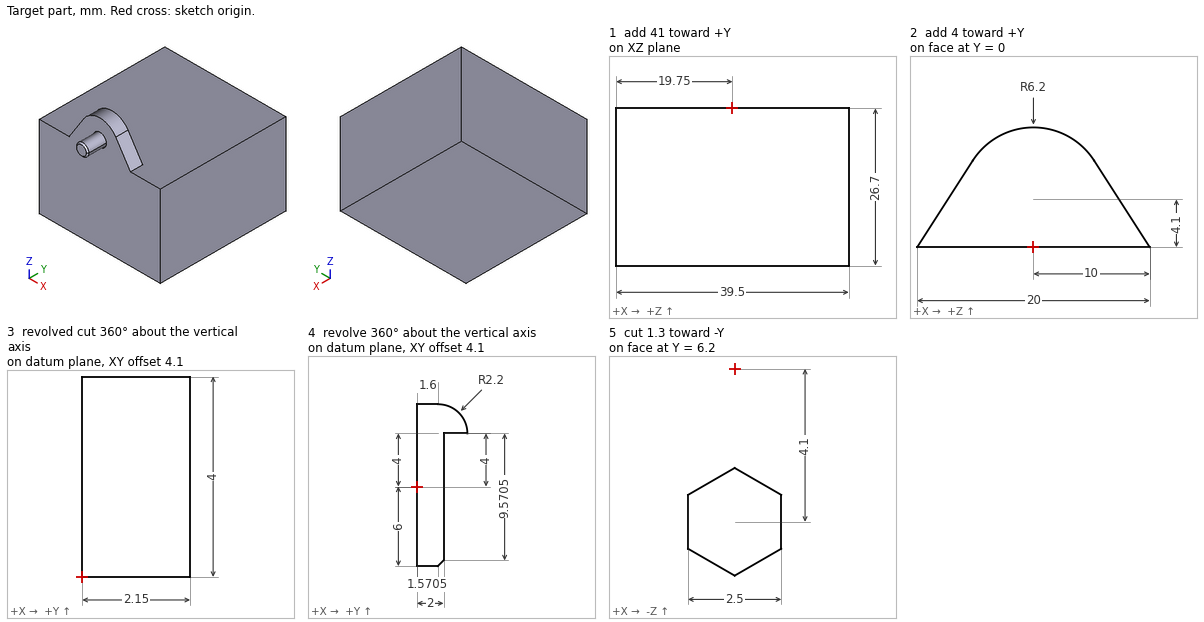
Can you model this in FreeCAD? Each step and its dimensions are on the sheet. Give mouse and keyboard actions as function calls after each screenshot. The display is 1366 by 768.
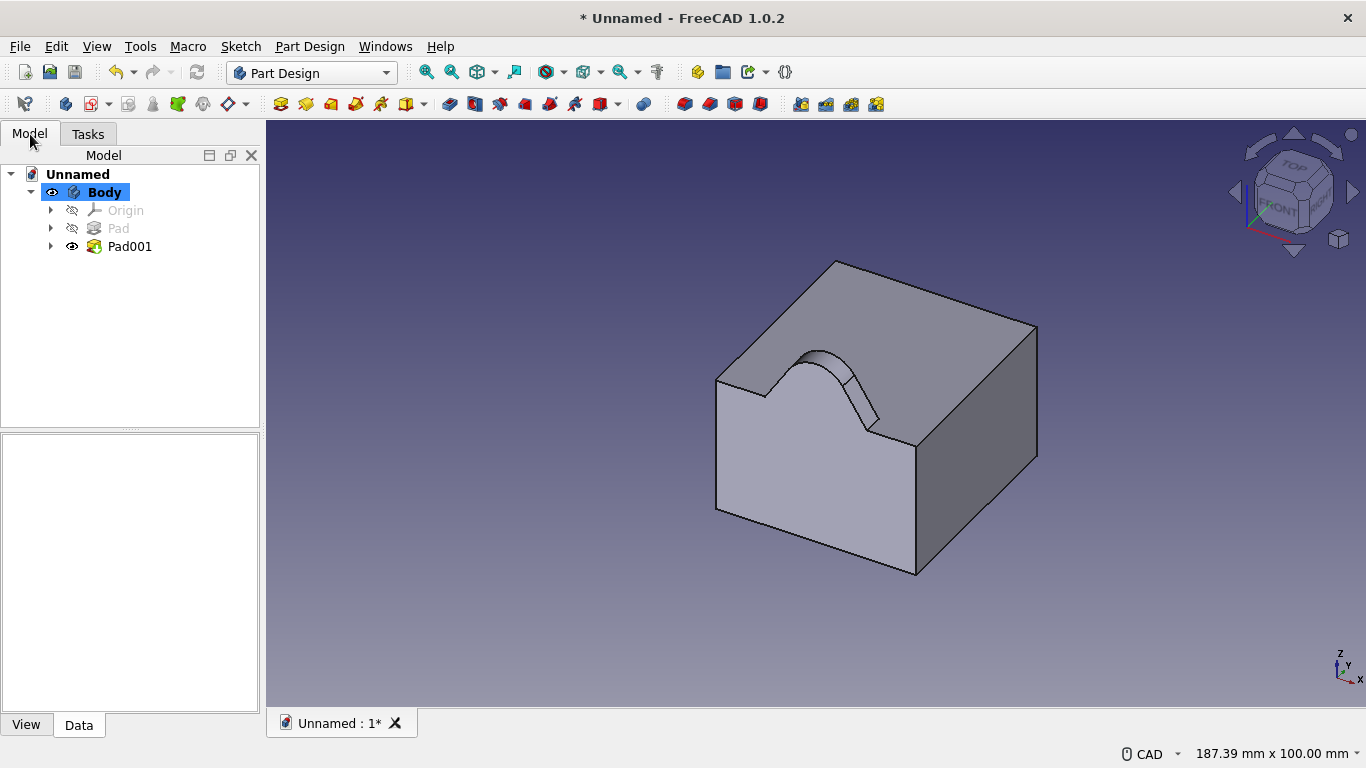
click(51, 210)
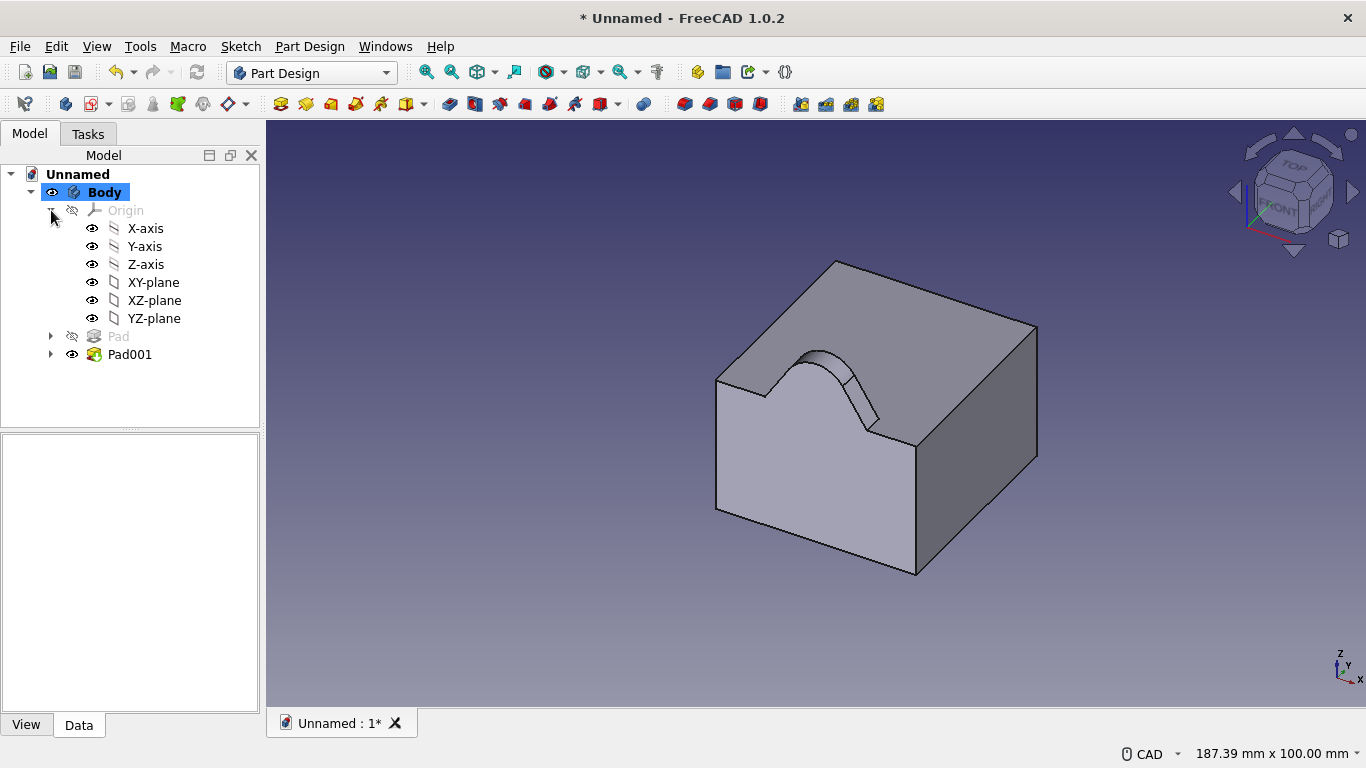
click(137, 282)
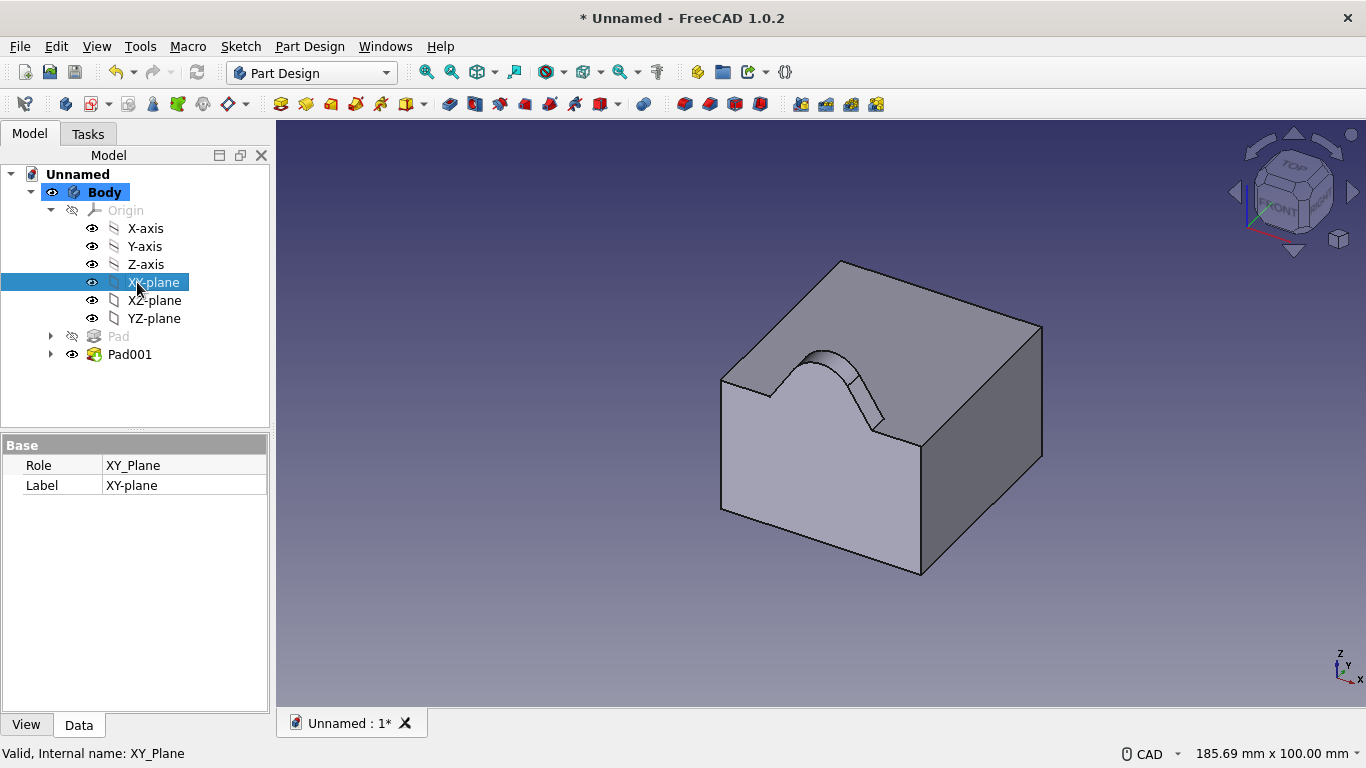
click(228, 104)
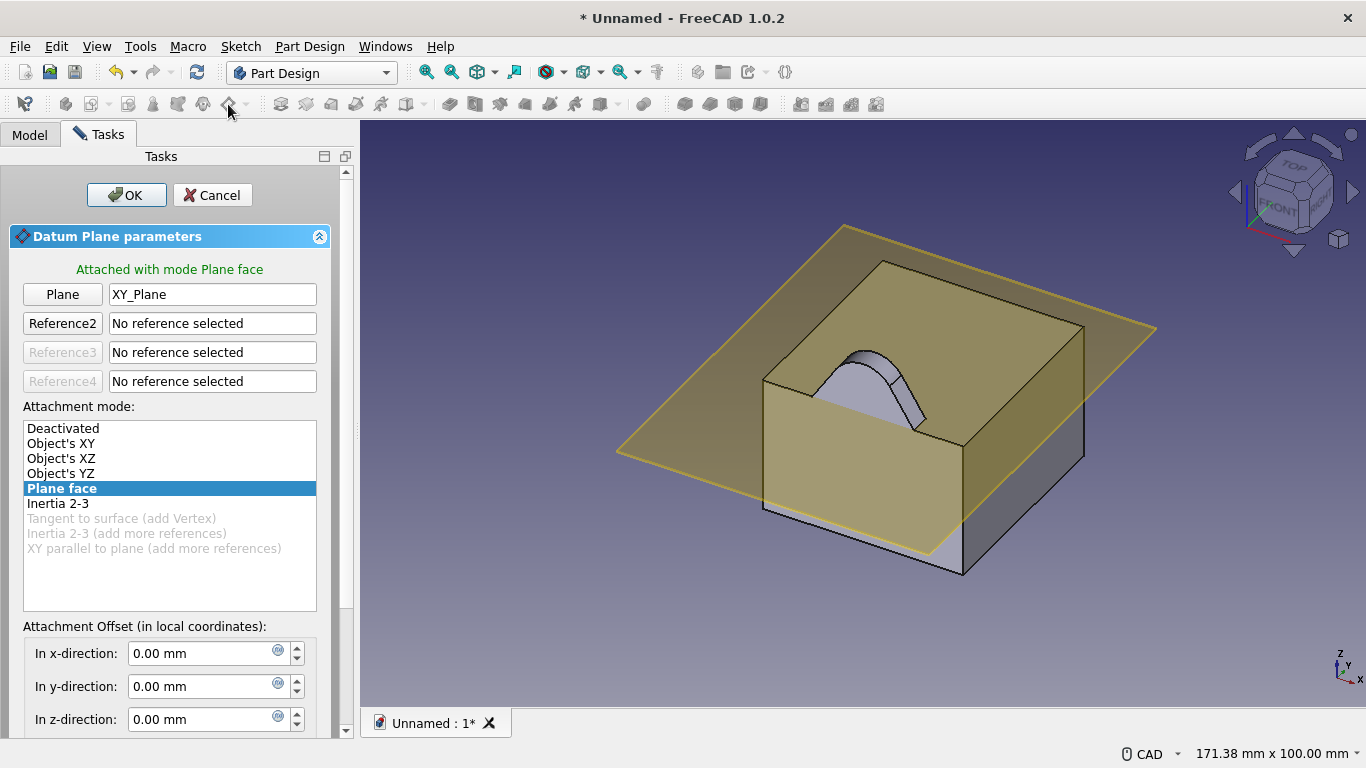
triple_click(210, 720)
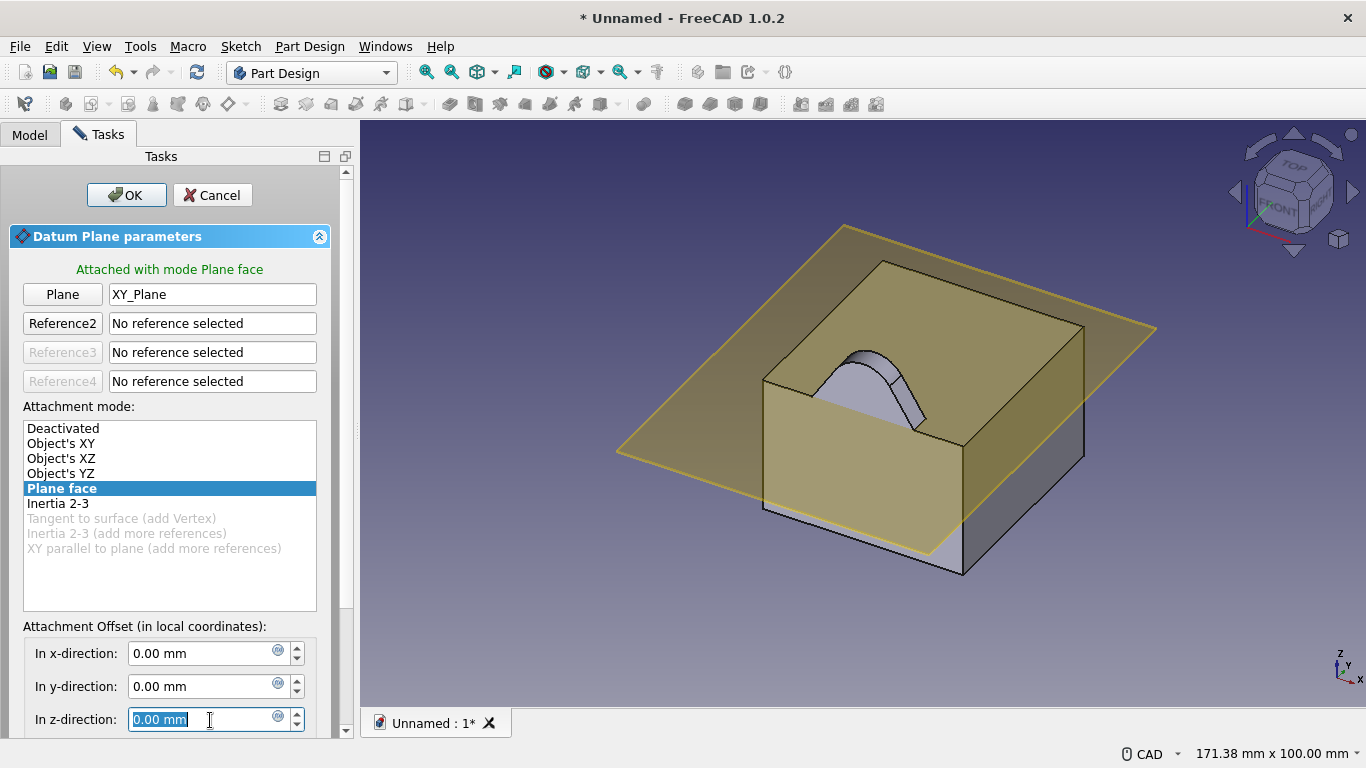
text(4.1)
key(Tab)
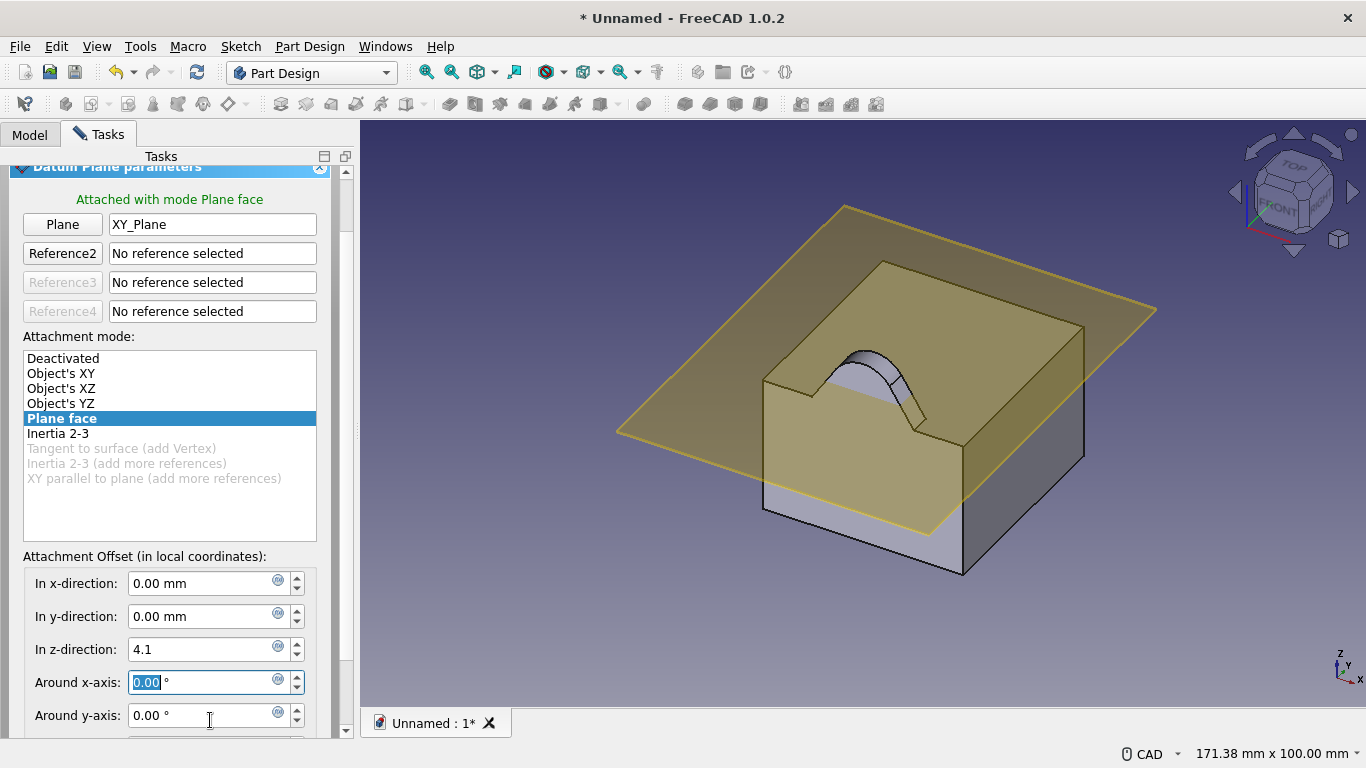
scroll(346, 452, up, 2)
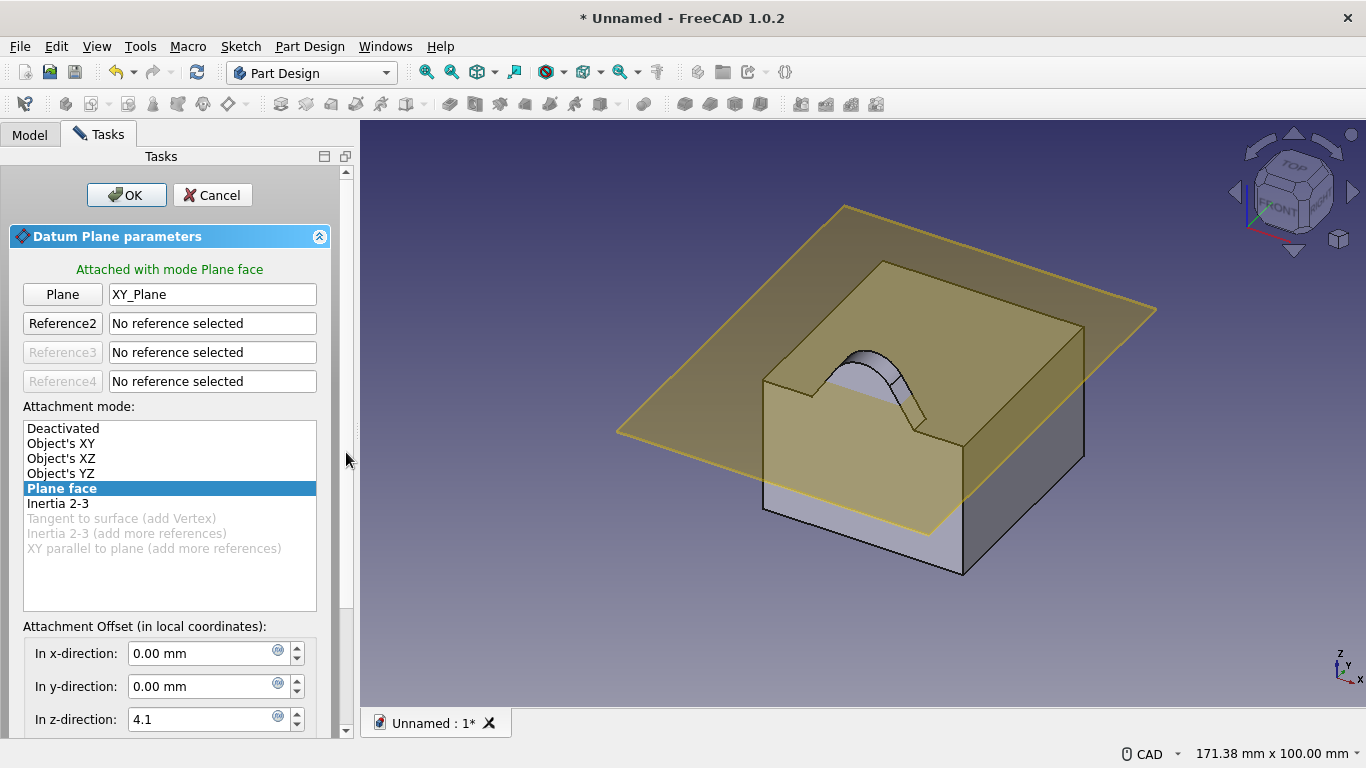
click(127, 195)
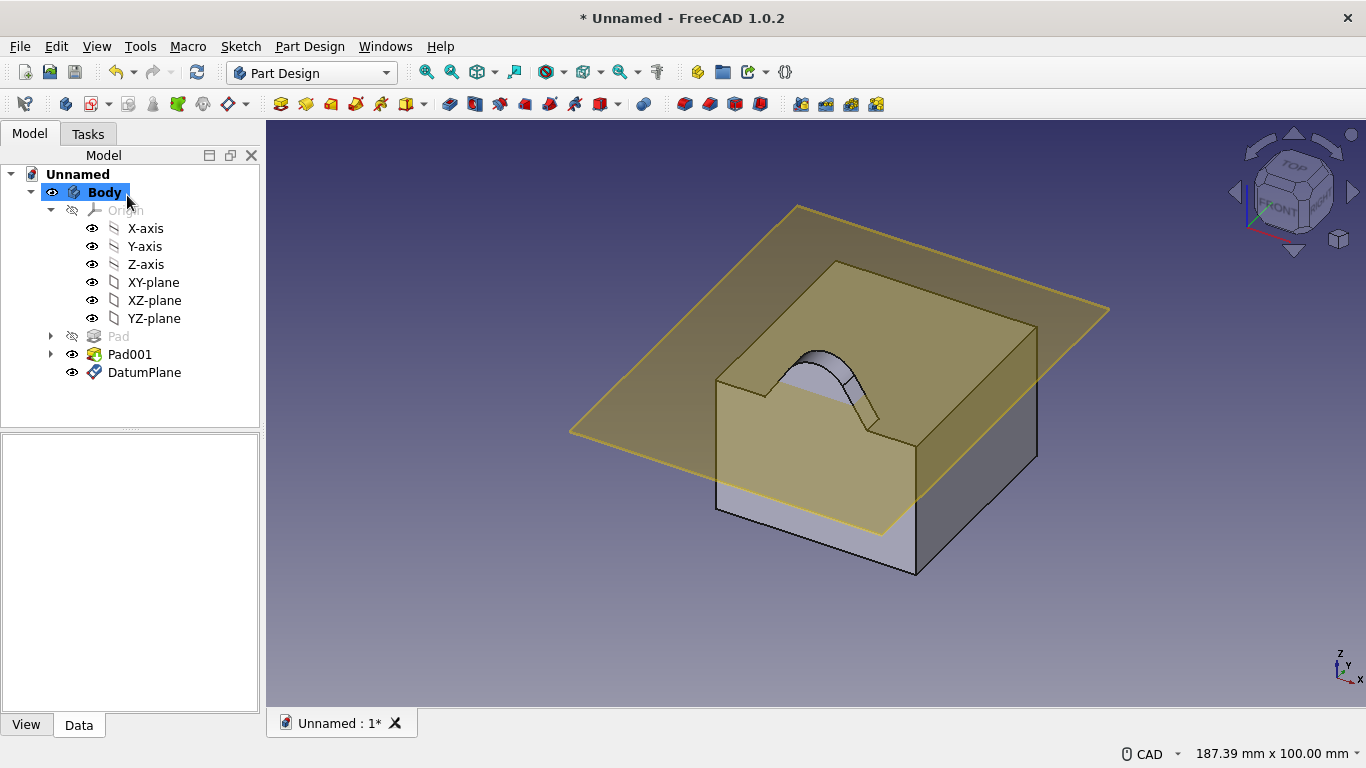
click(117, 372)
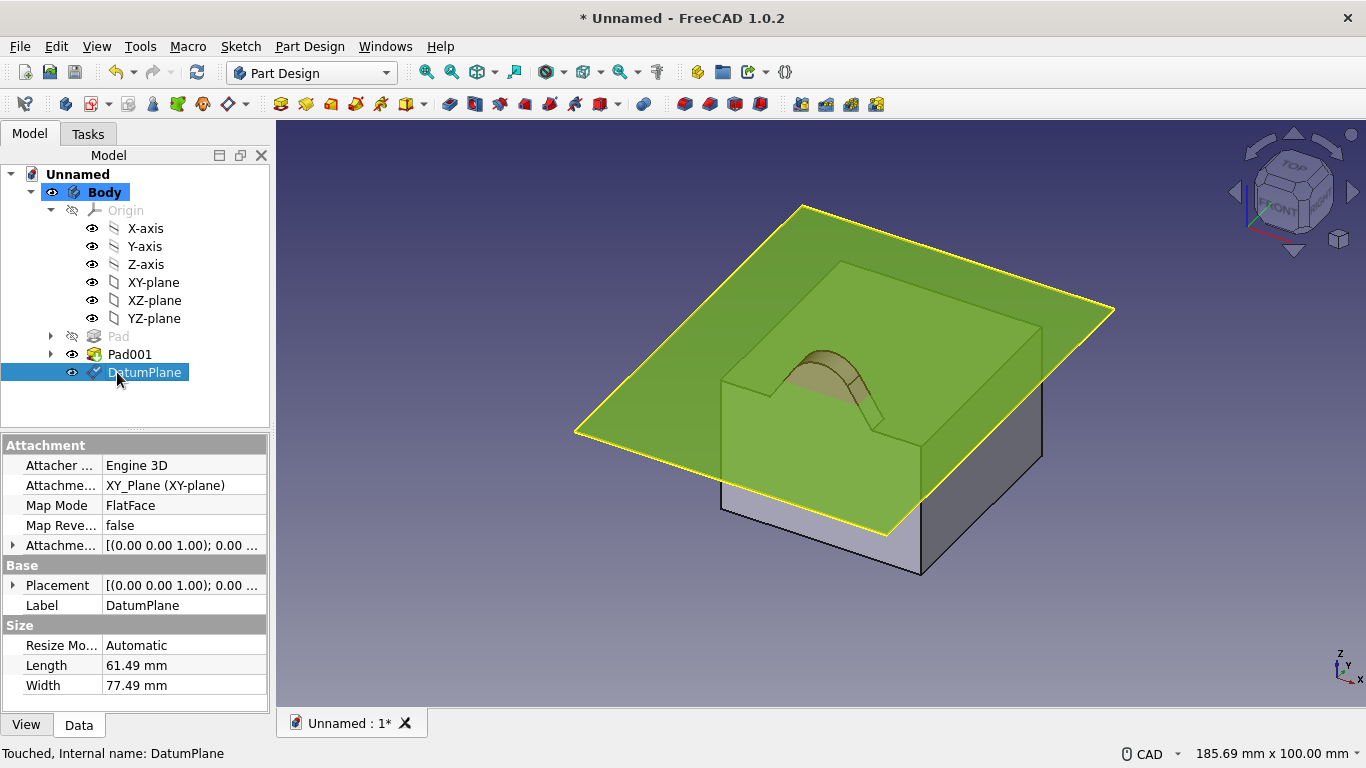
click(90, 104)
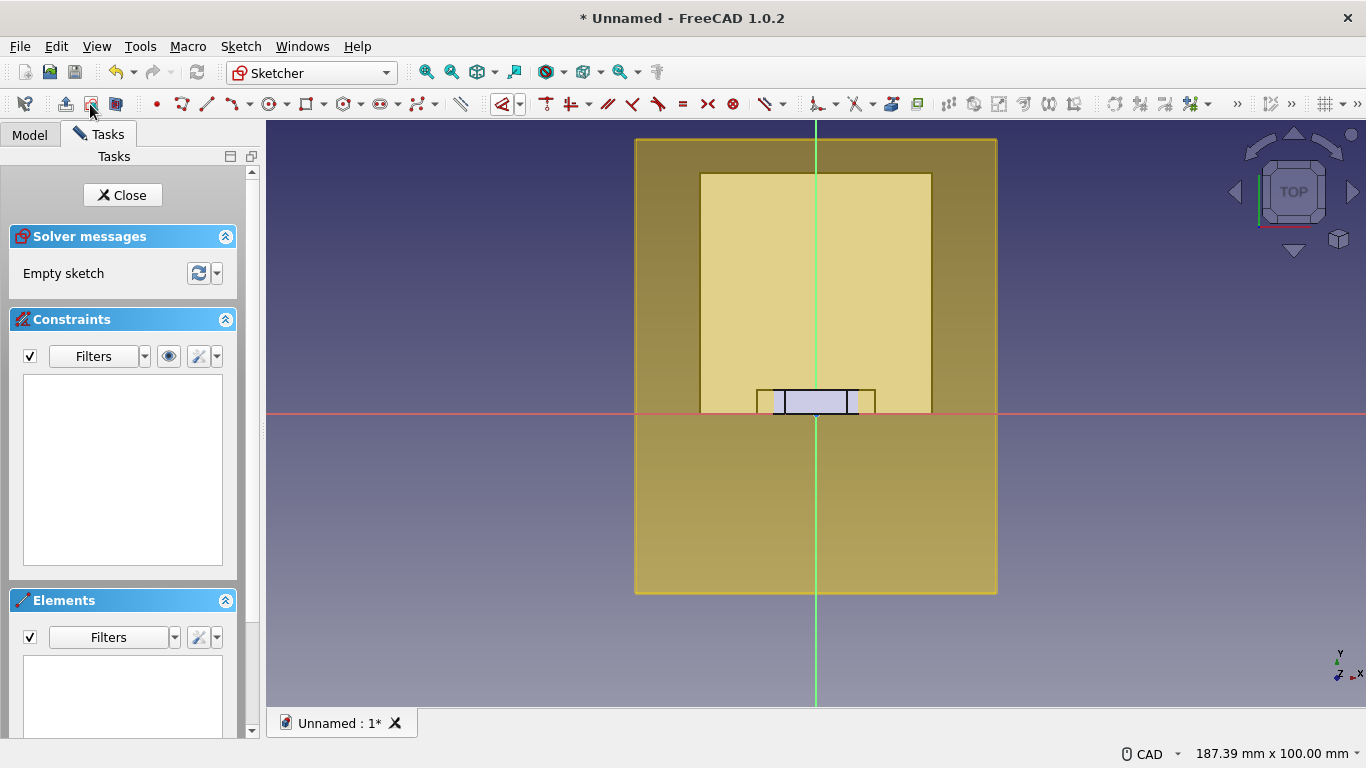
key(q)
key(s)